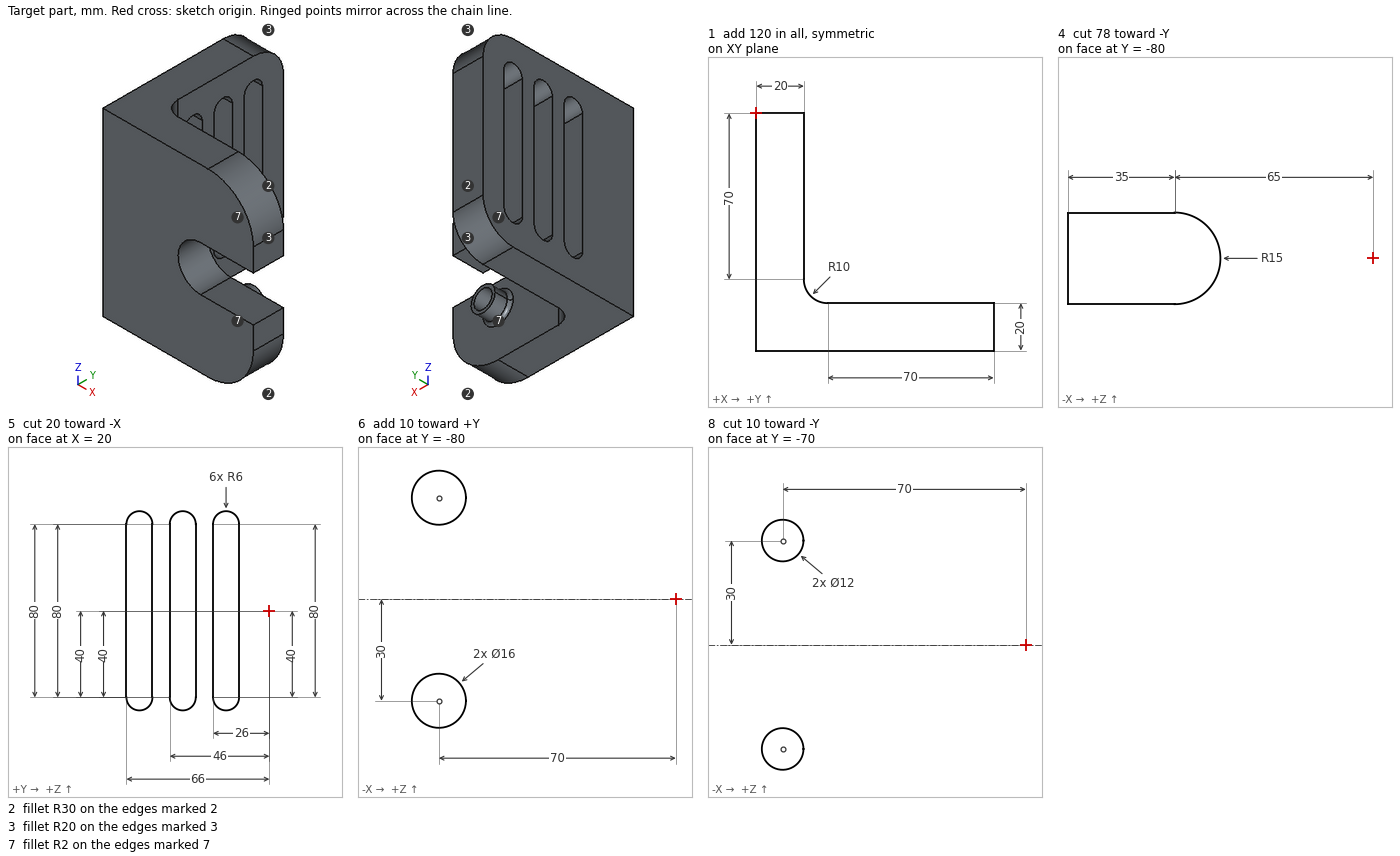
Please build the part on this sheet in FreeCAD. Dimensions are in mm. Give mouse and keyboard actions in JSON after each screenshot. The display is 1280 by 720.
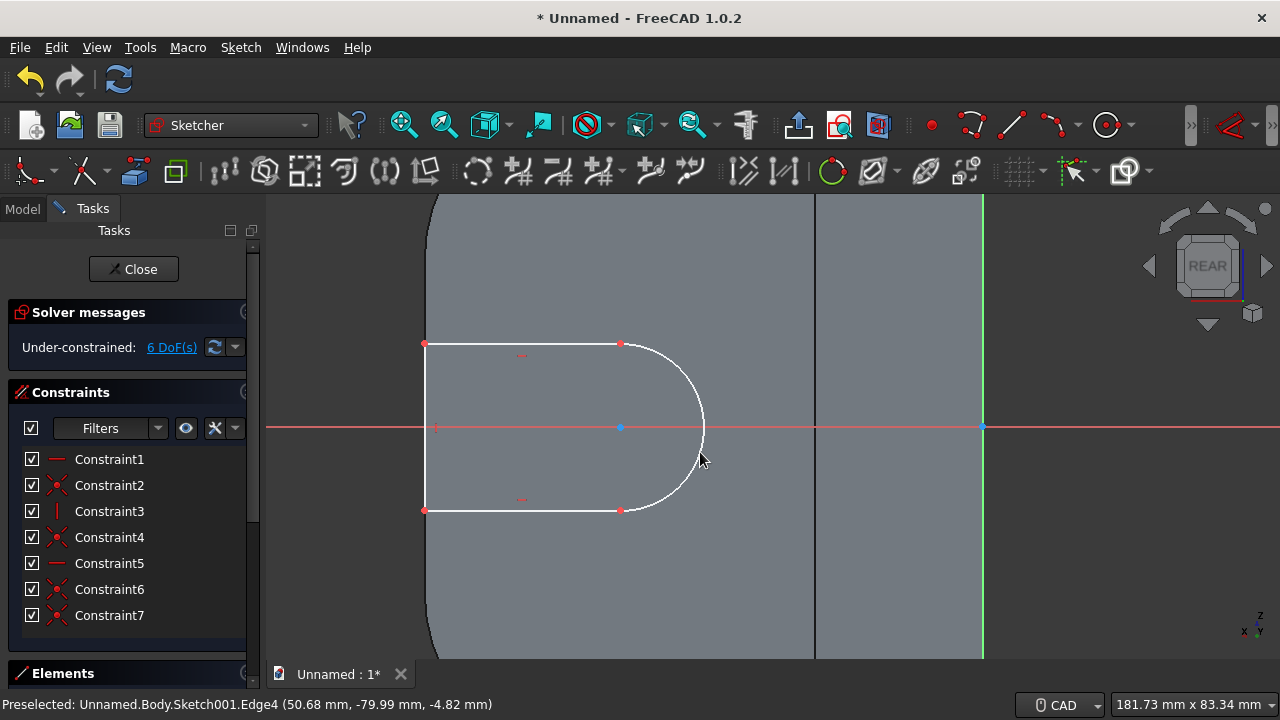
{"action": "left_click", "coordinate": [562, 344]}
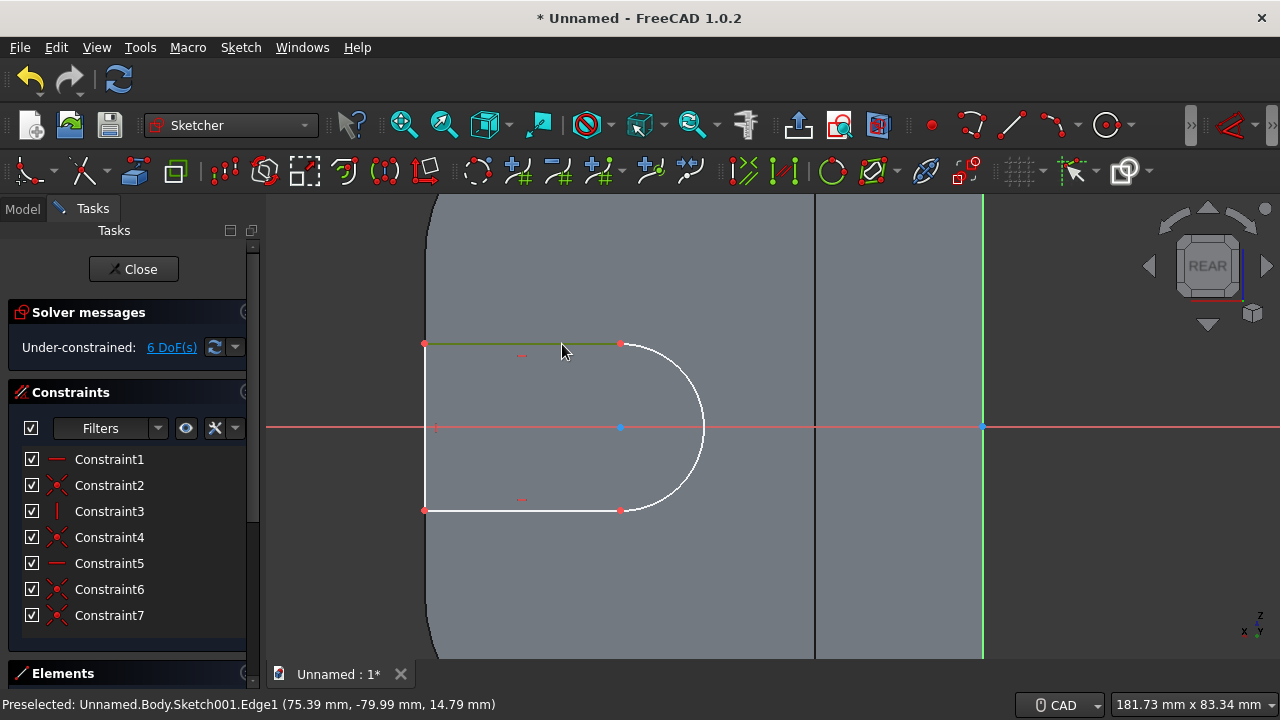
{"action": "left_click", "coordinate": [688, 477]}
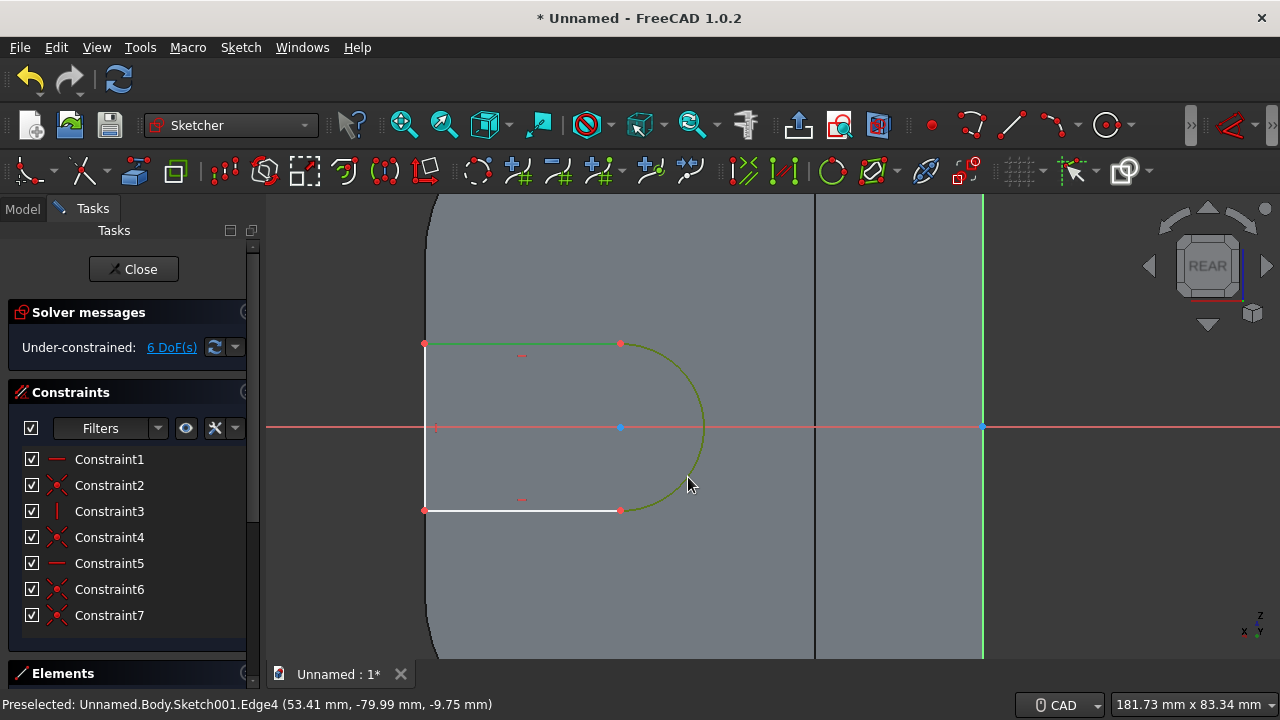
{"action": "key", "text": "t"}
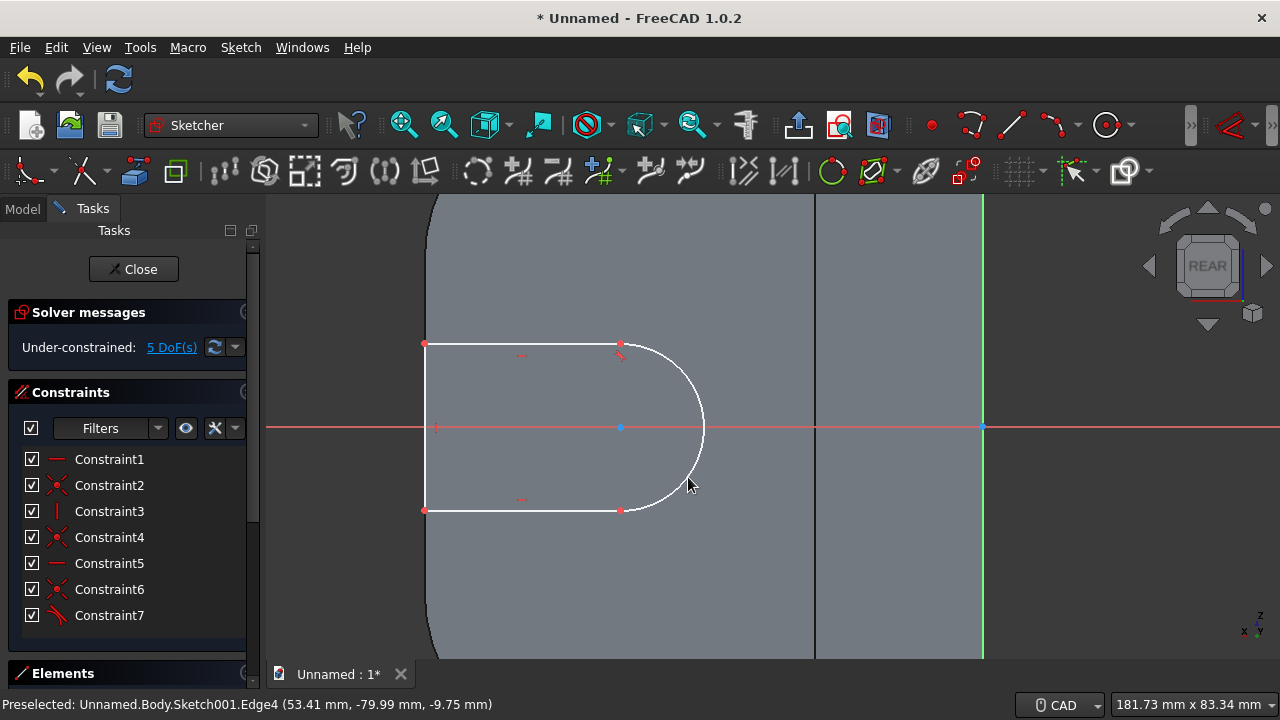
{"action": "left_click", "coordinate": [484, 511]}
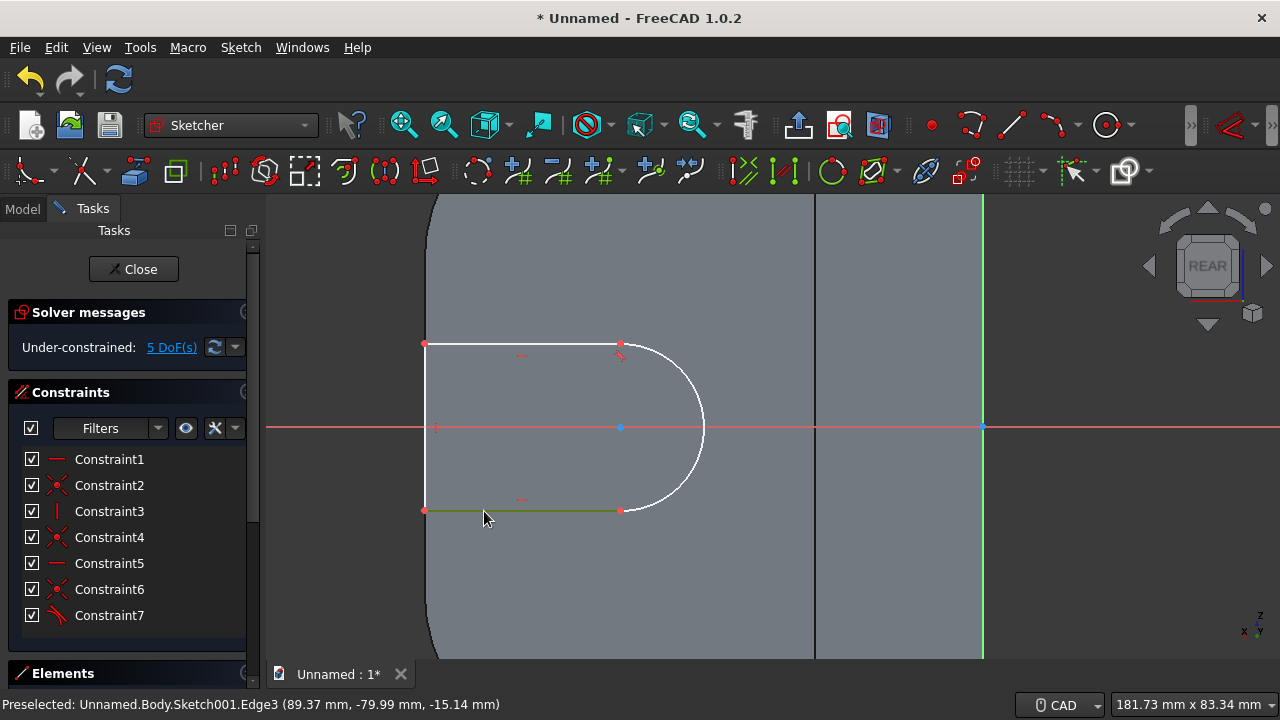
{"action": "left_click", "coordinate": [688, 477]}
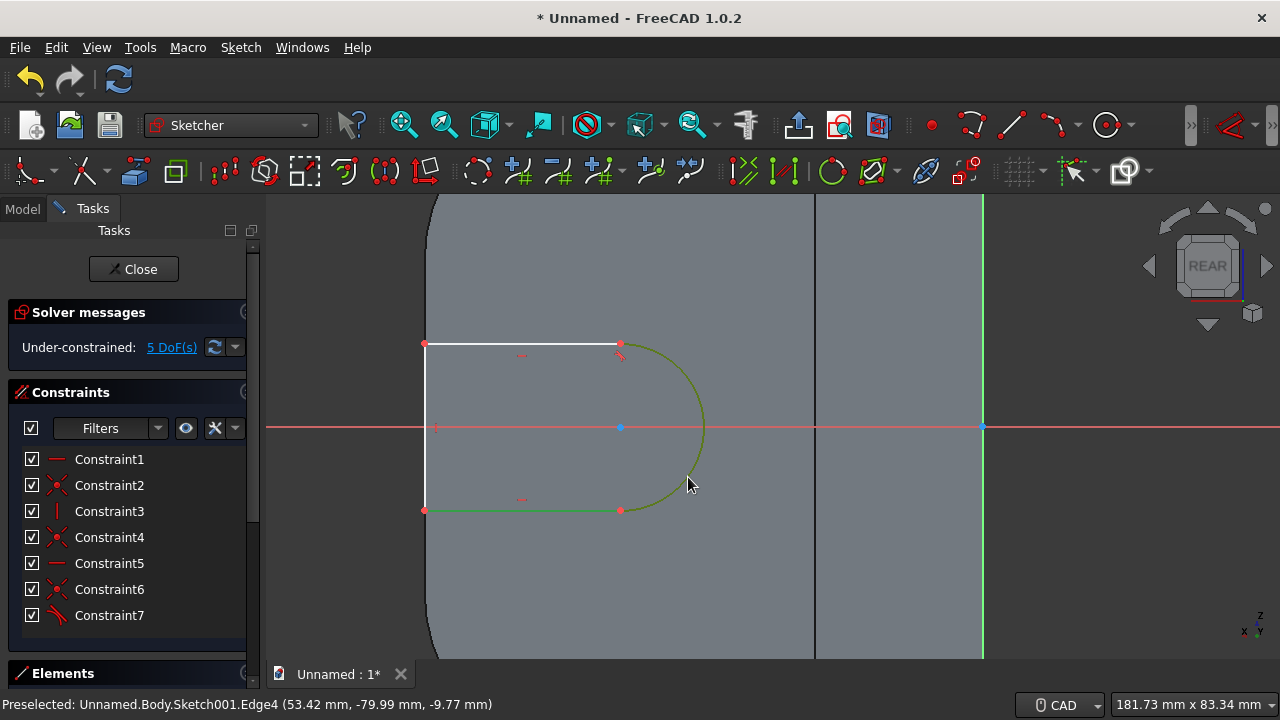
{"action": "key", "text": "t"}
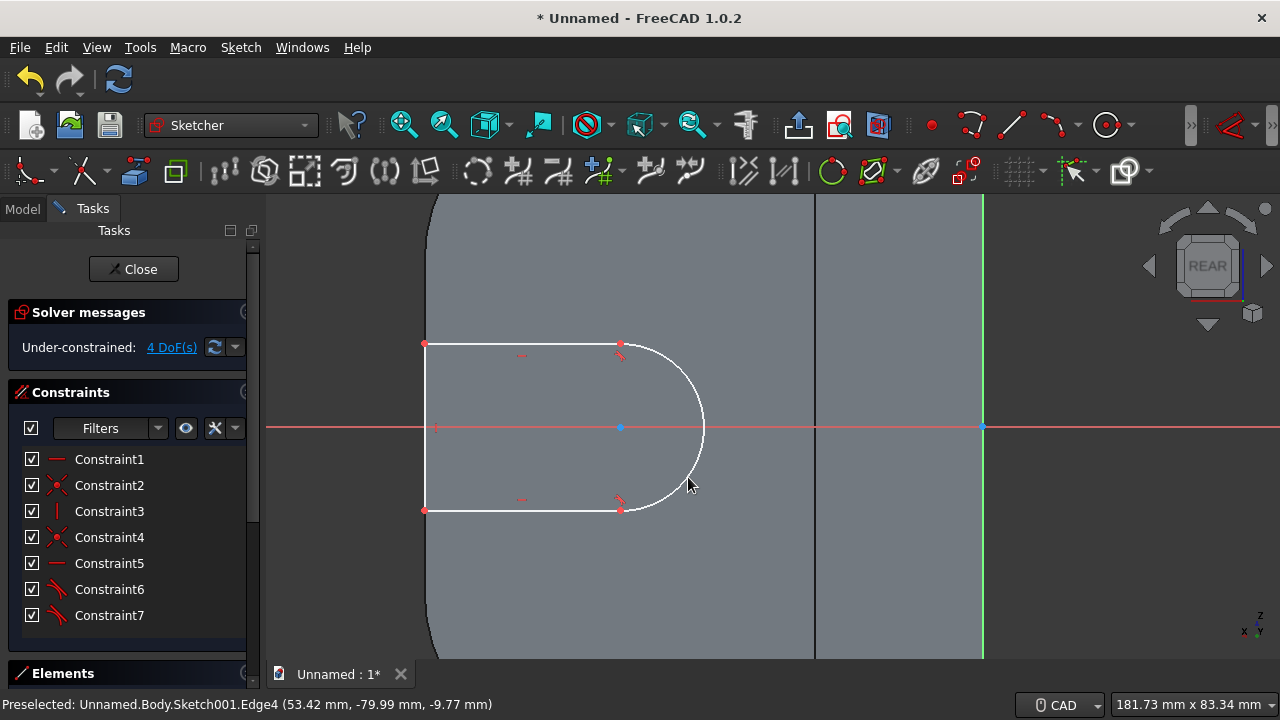
{"action": "left_click", "coordinate": [620, 427]}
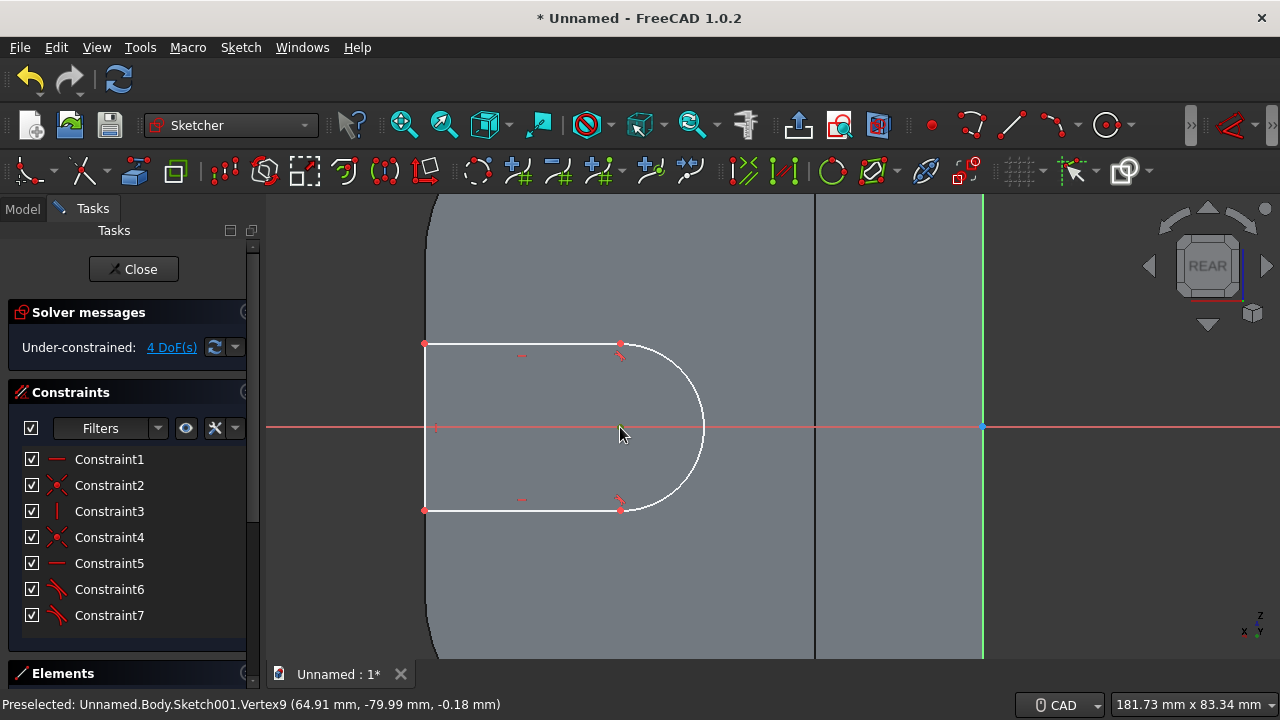
{"action": "left_click", "coordinate": [353, 426]}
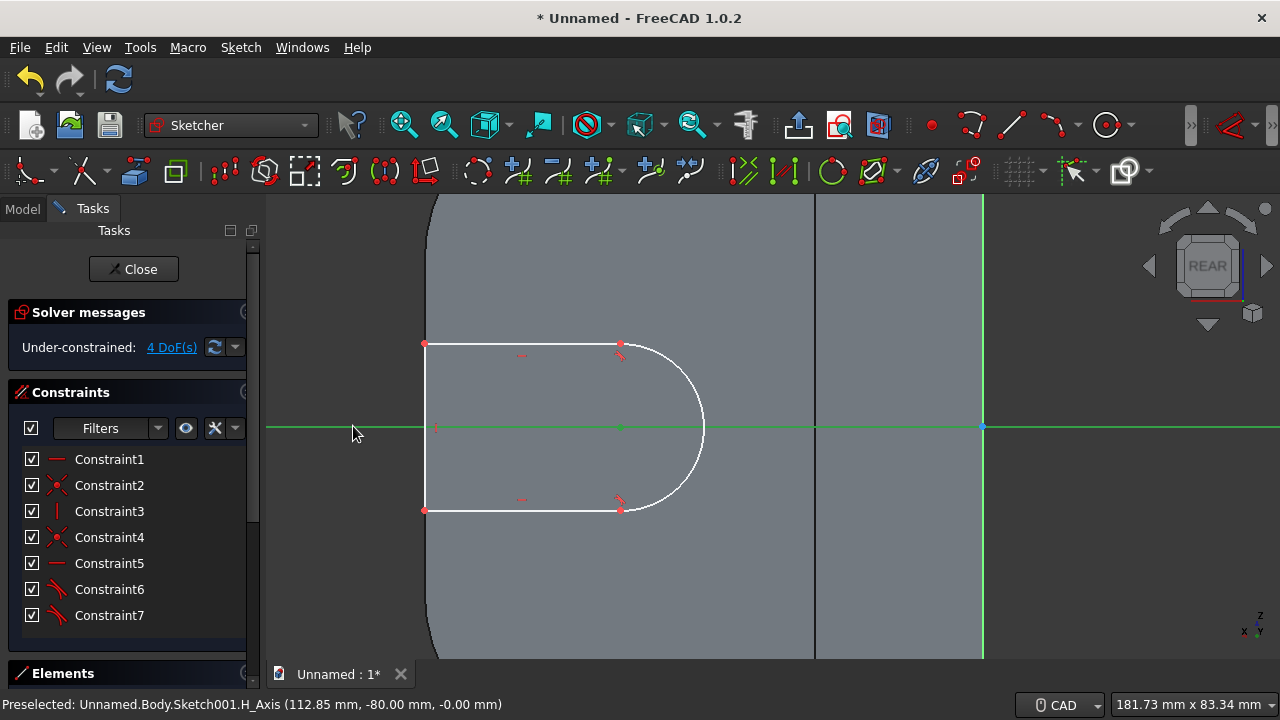
{"action": "key", "text": "c"}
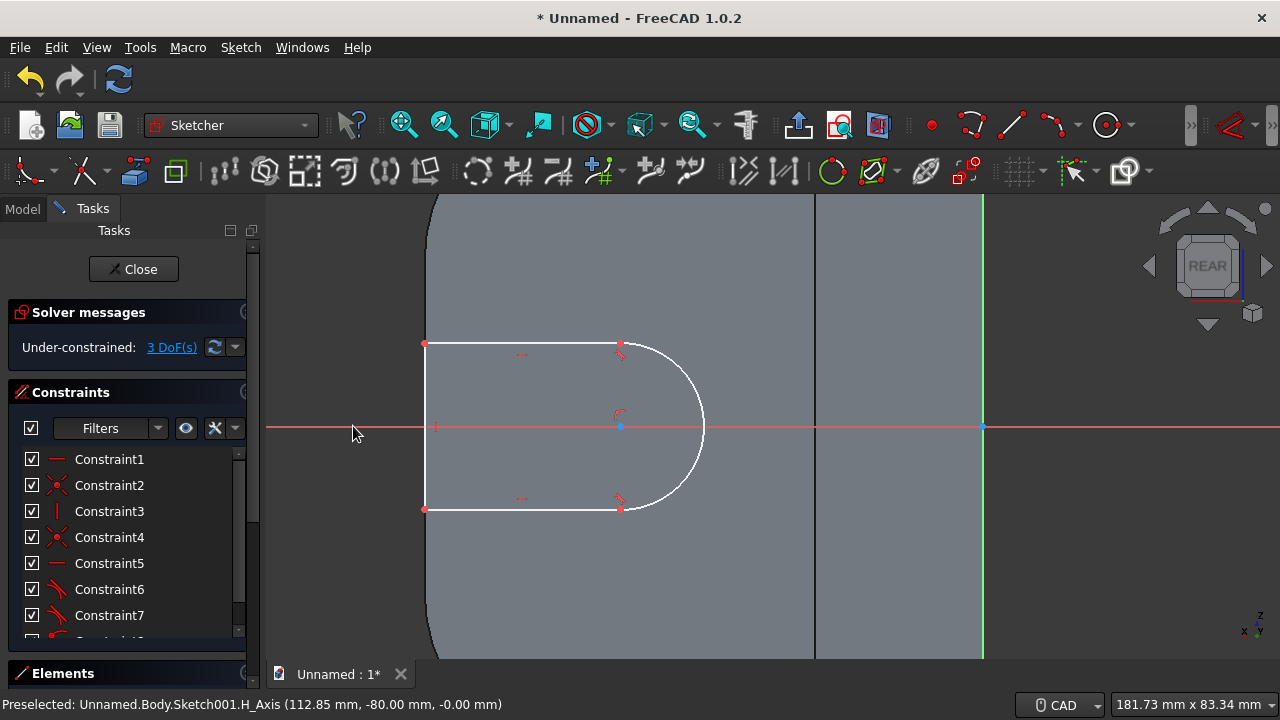
{"action": "key", "text": "d"}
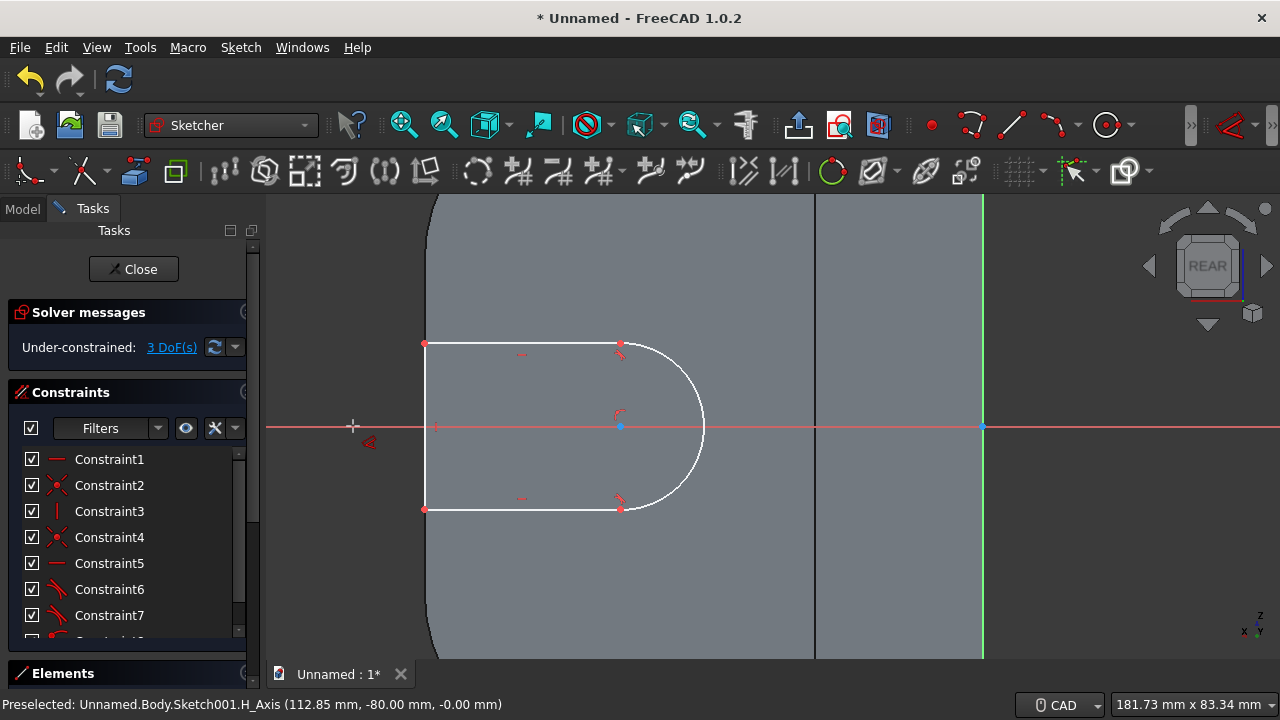
{"action": "left_click", "coordinate": [688, 476]}
{"action": "left_click", "coordinate": [714, 495]}